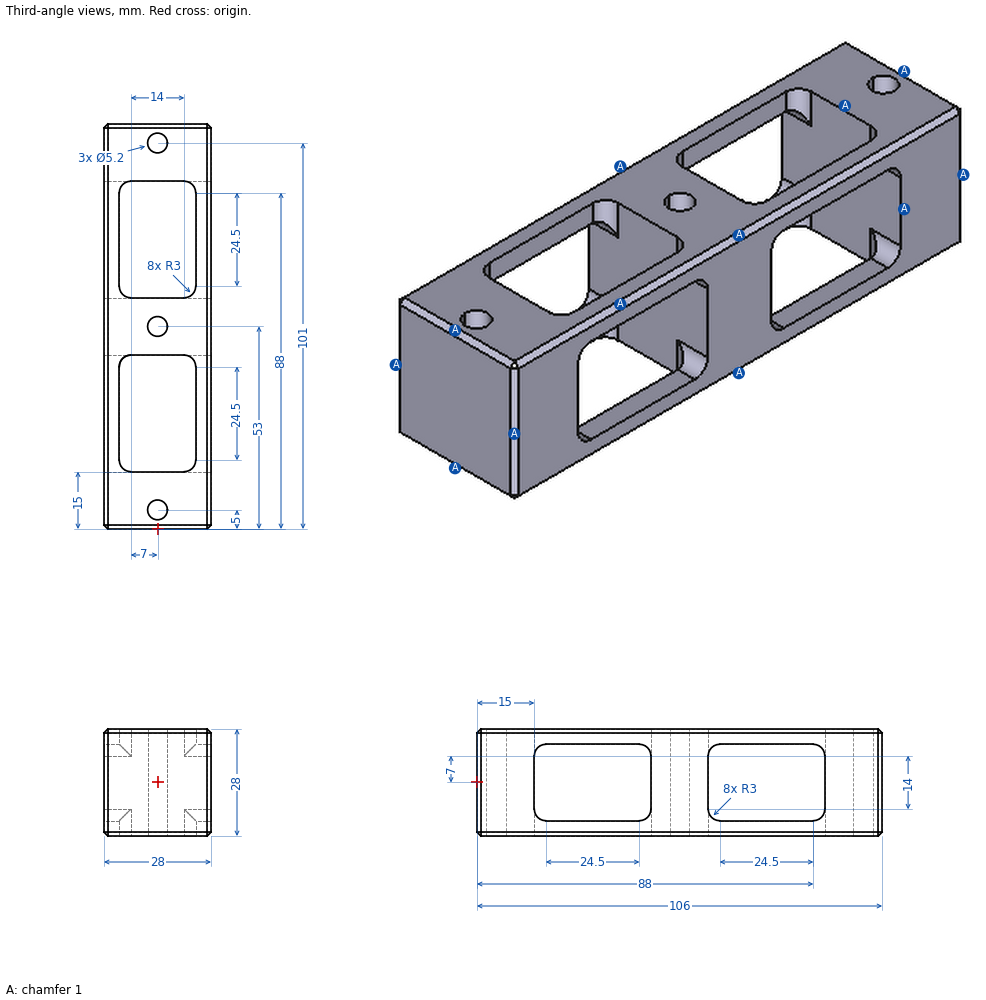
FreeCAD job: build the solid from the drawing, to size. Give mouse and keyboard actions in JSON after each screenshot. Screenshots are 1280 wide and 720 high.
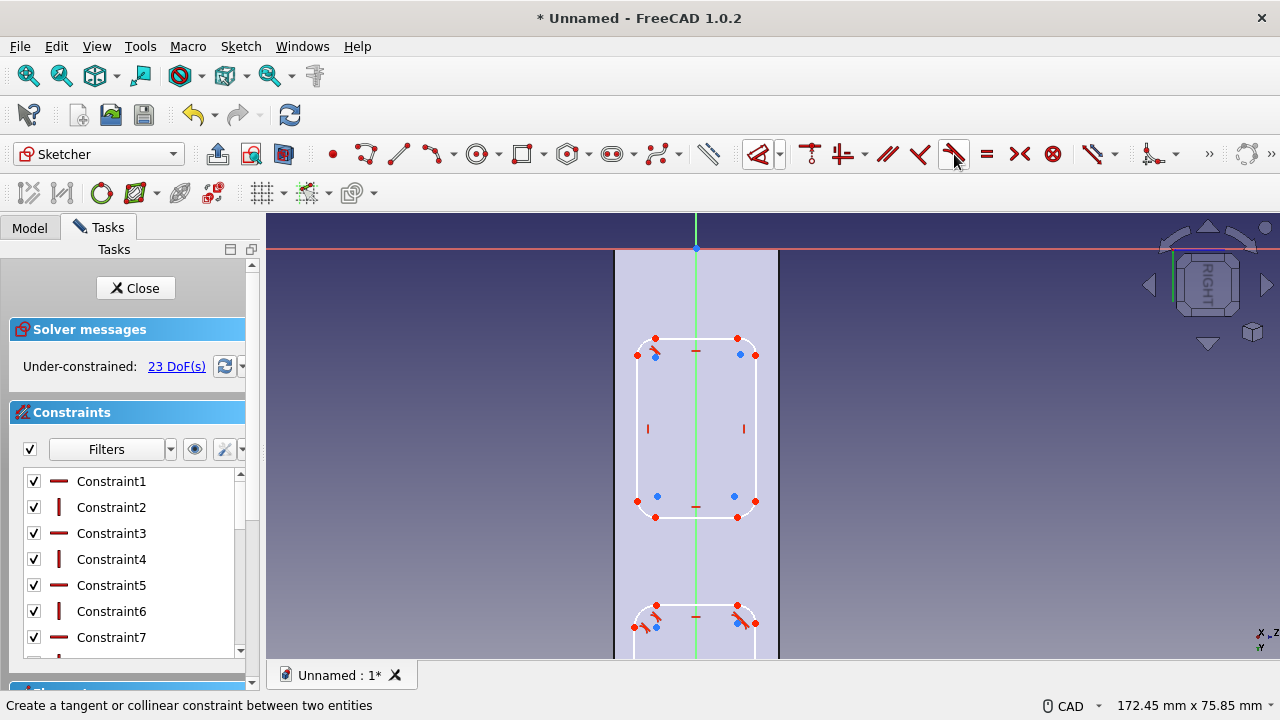
{"action": "left_click", "coordinate": [713, 339]}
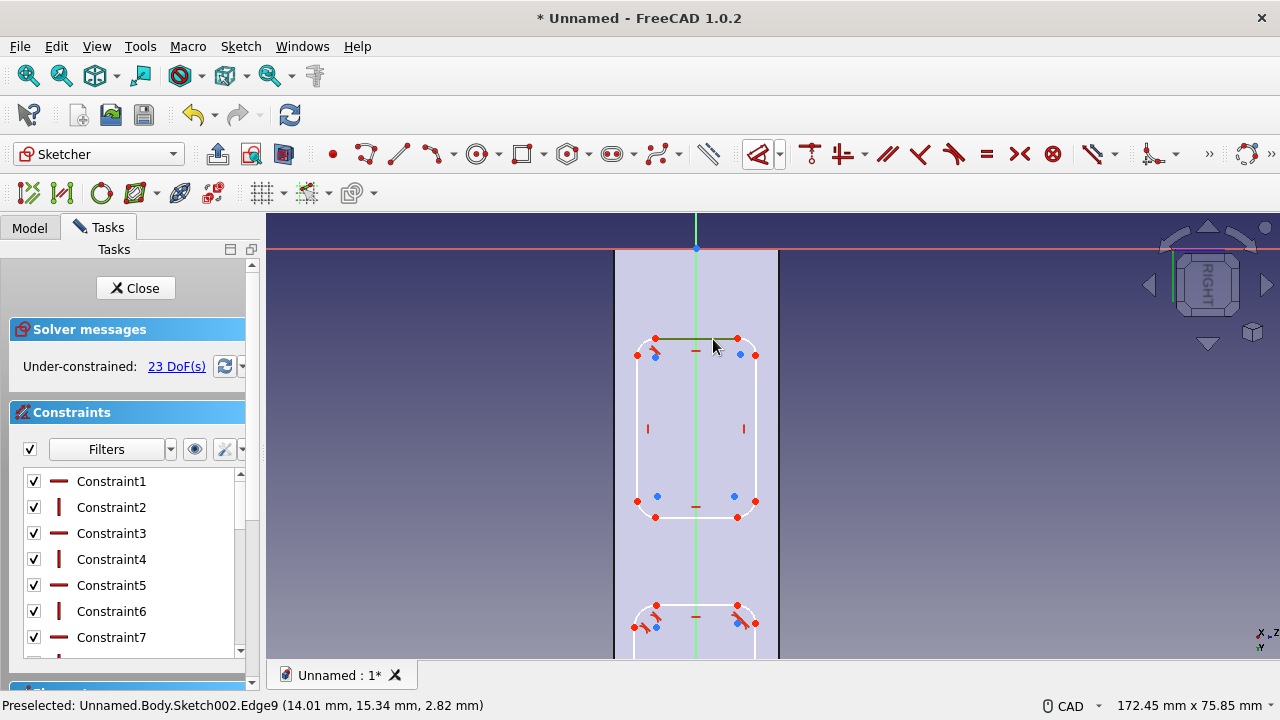
{"action": "left_click", "coordinate": [751, 343]}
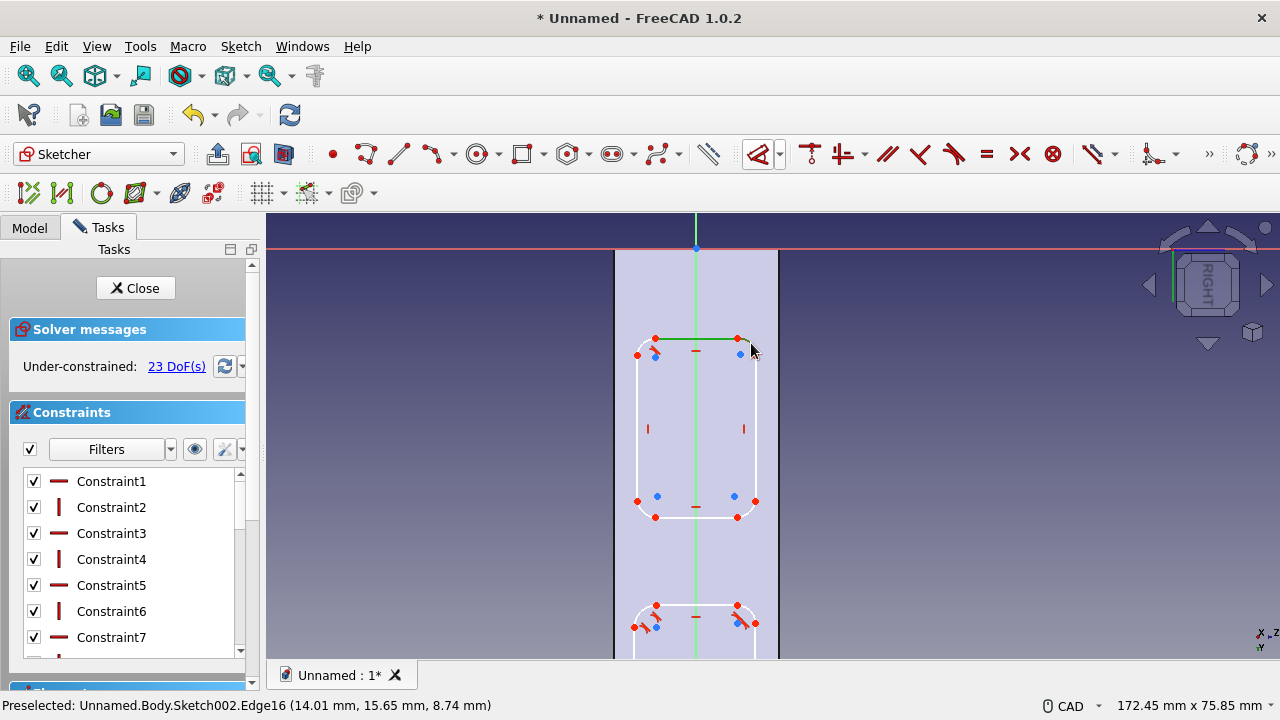
{"action": "left_click", "coordinate": [954, 154]}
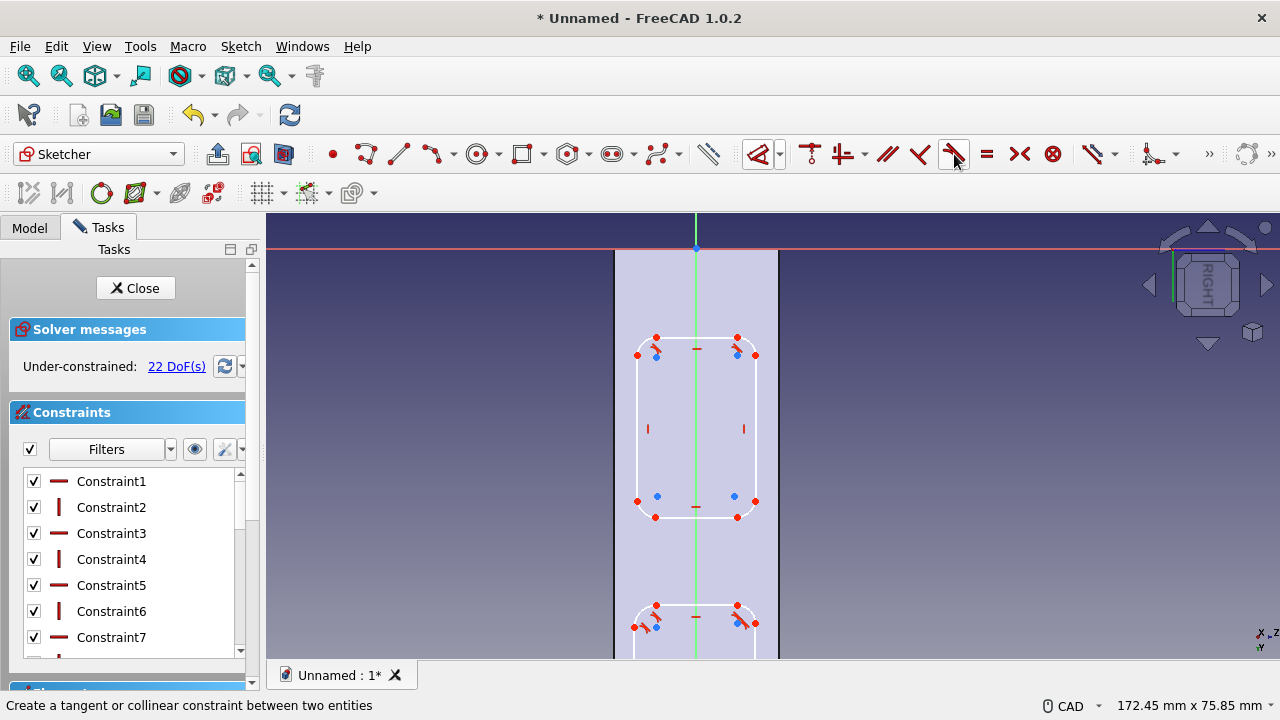
{"action": "left_click", "coordinate": [637, 399]}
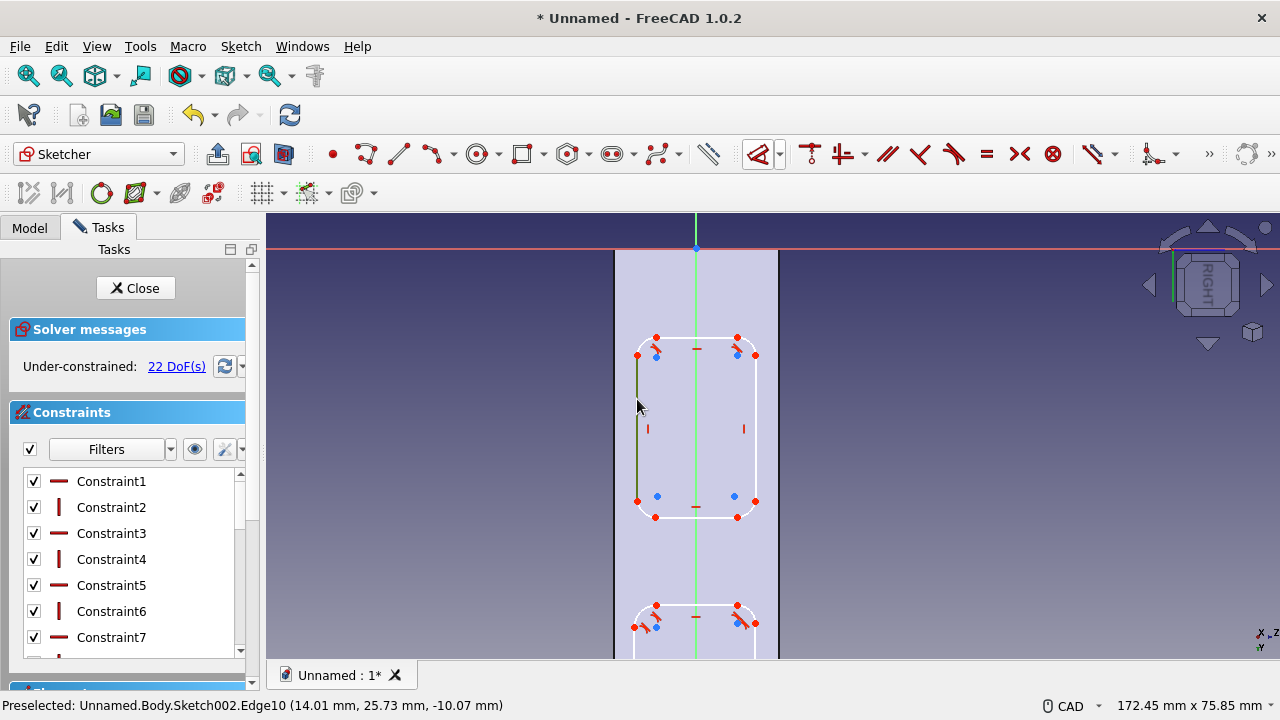
{"action": "left_click", "coordinate": [643, 343]}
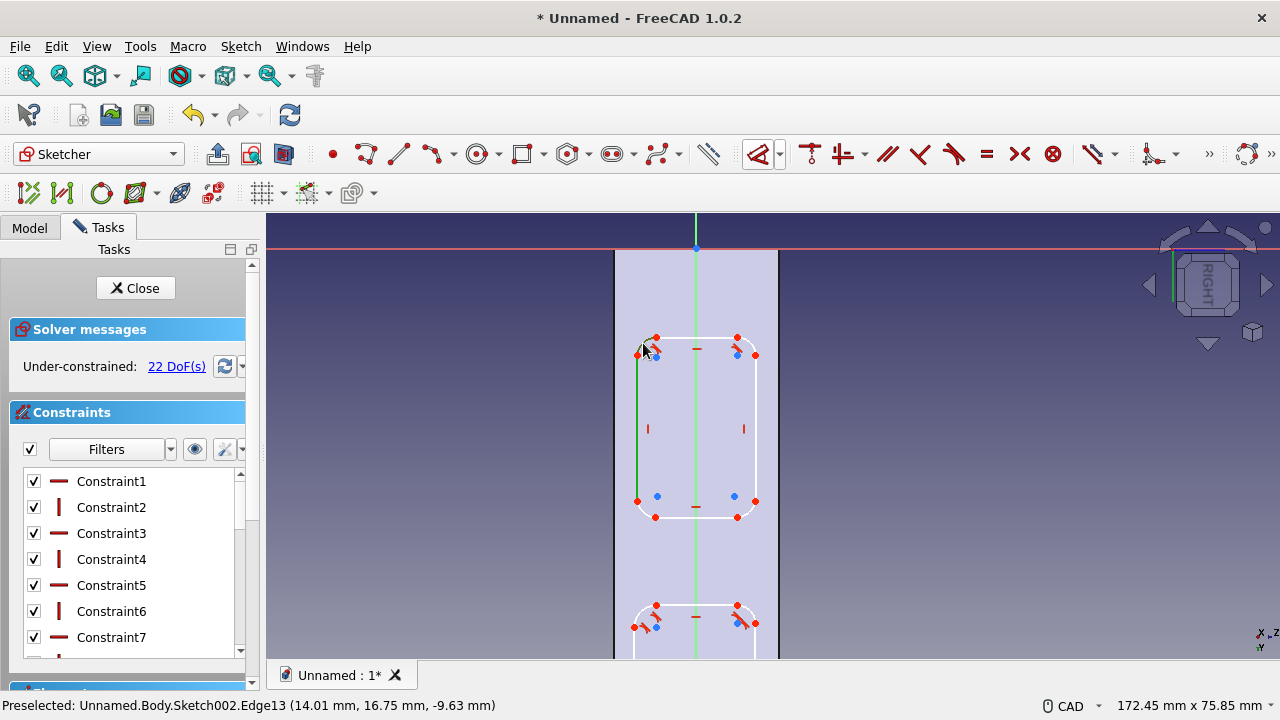
{"action": "left_click", "coordinate": [954, 154]}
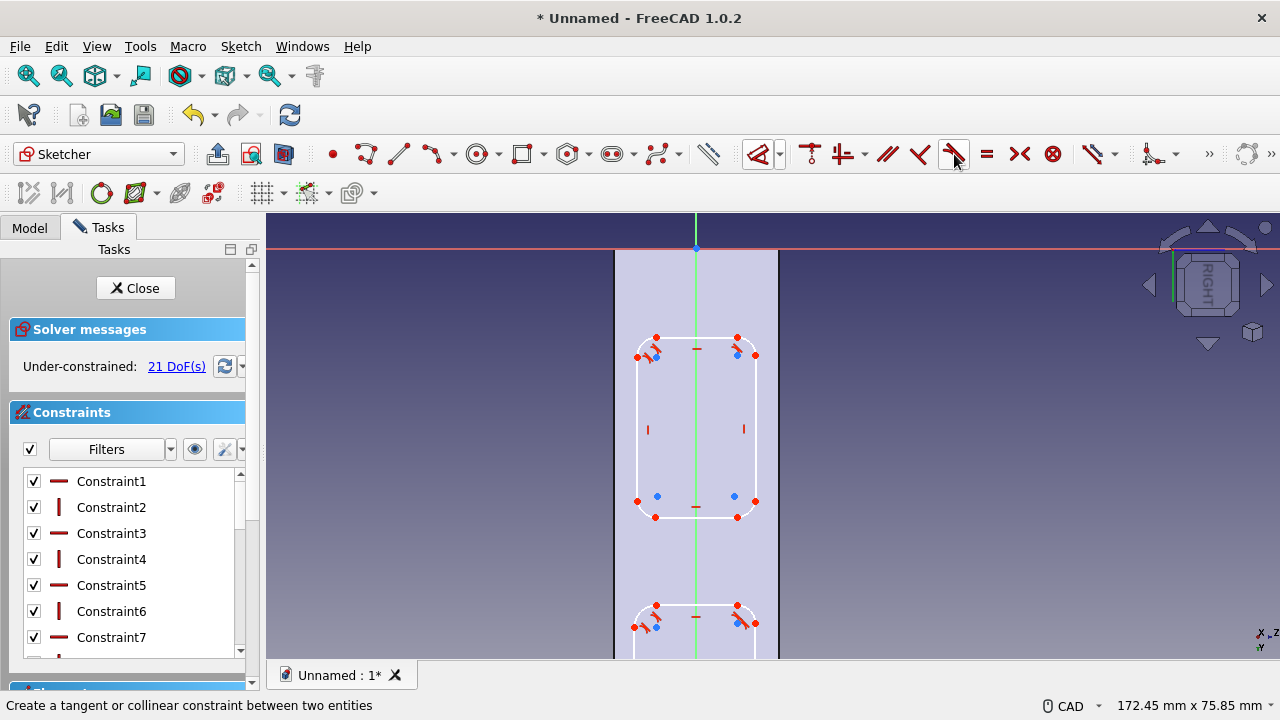
{"action": "left_click", "coordinate": [637, 400]}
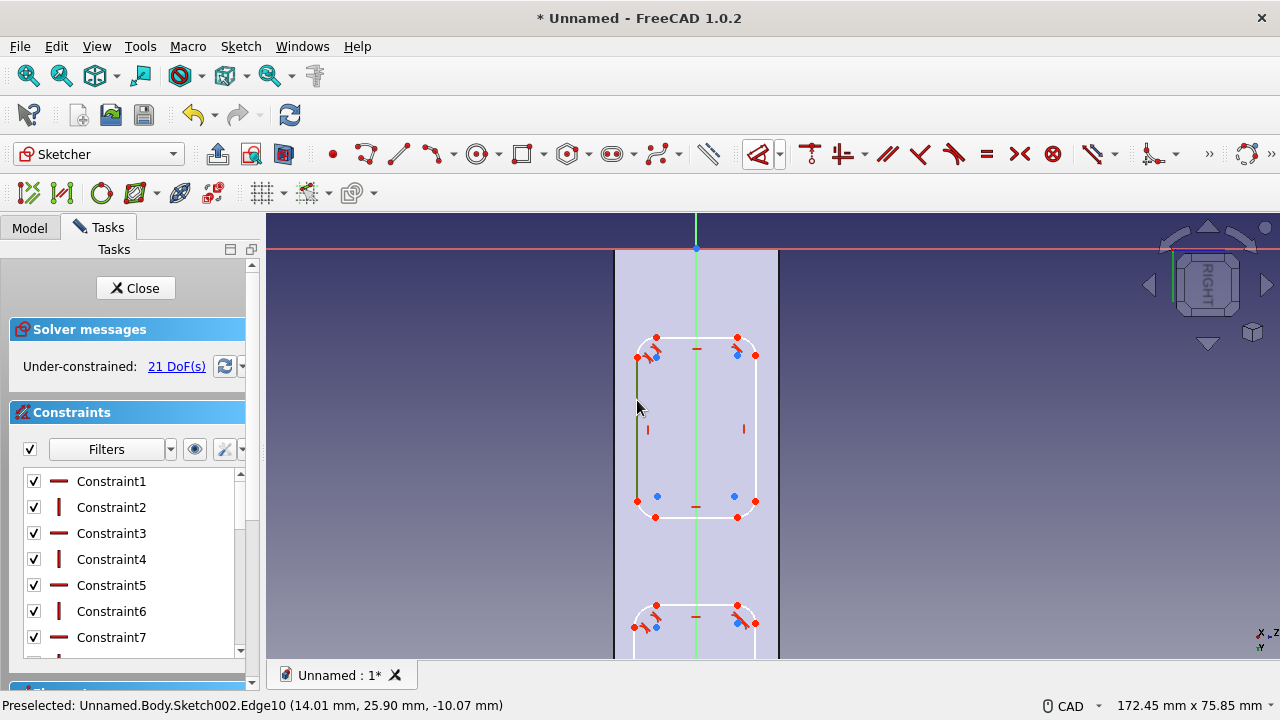
{"action": "left_click", "coordinate": [644, 512]}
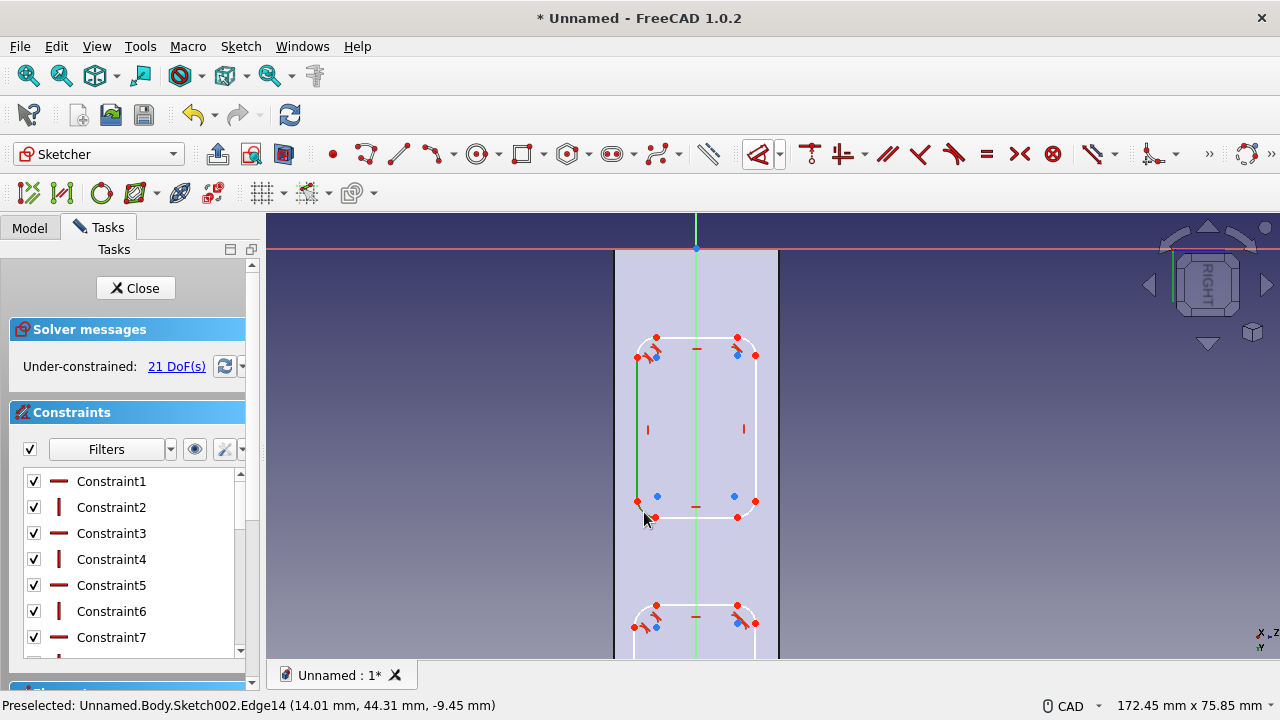
{"action": "left_click", "coordinate": [954, 154]}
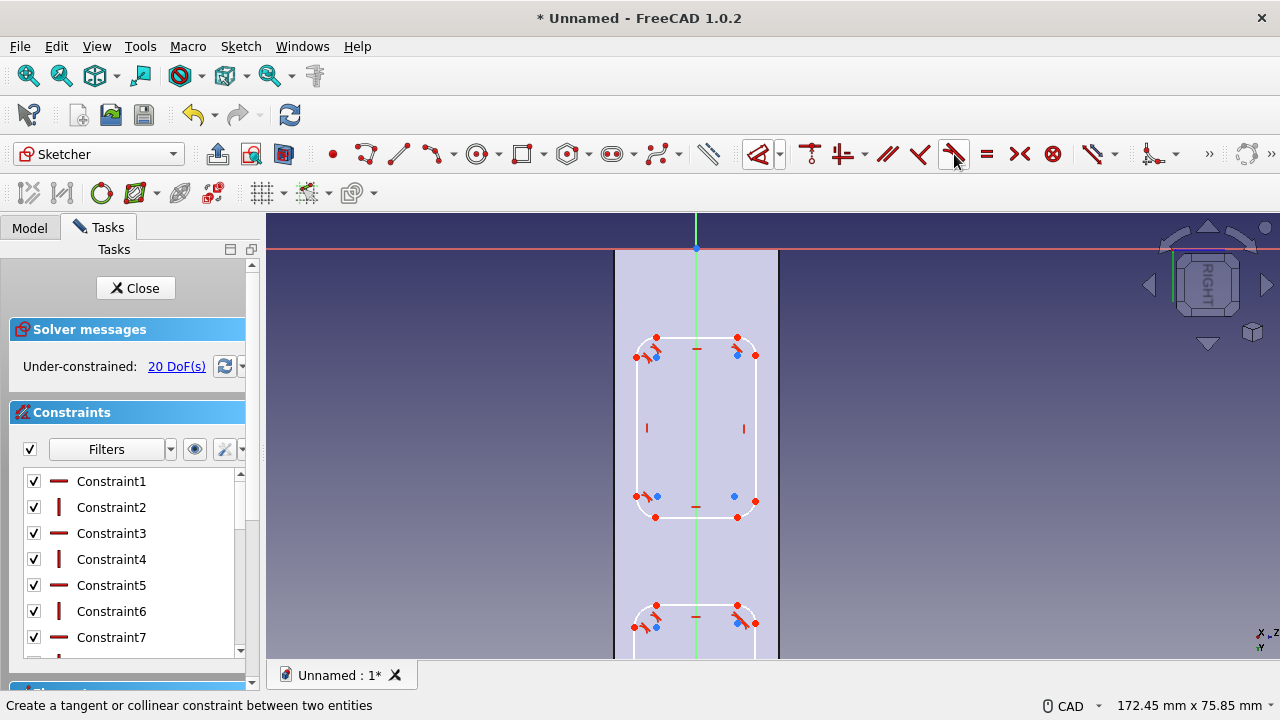
{"action": "left_click", "coordinate": [680, 518]}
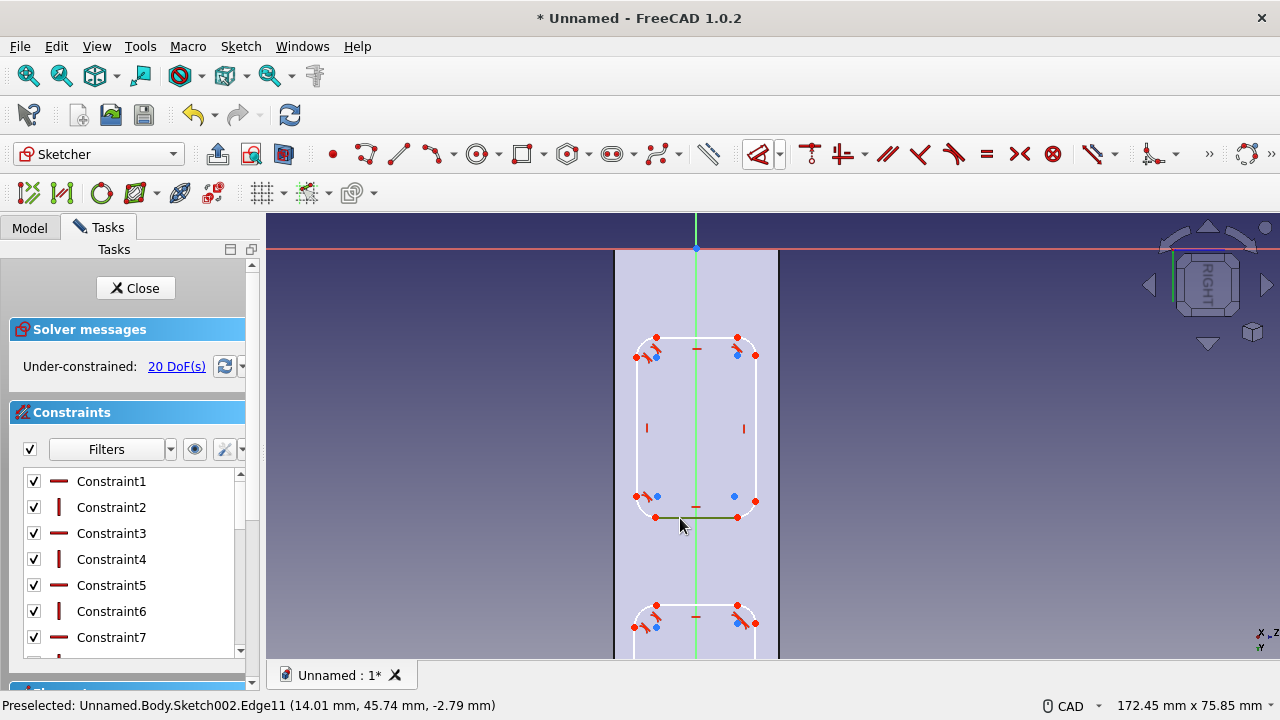
{"action": "scroll", "coordinate": [639, 506], "scroll_direction": "up", "scroll_amount": 3}